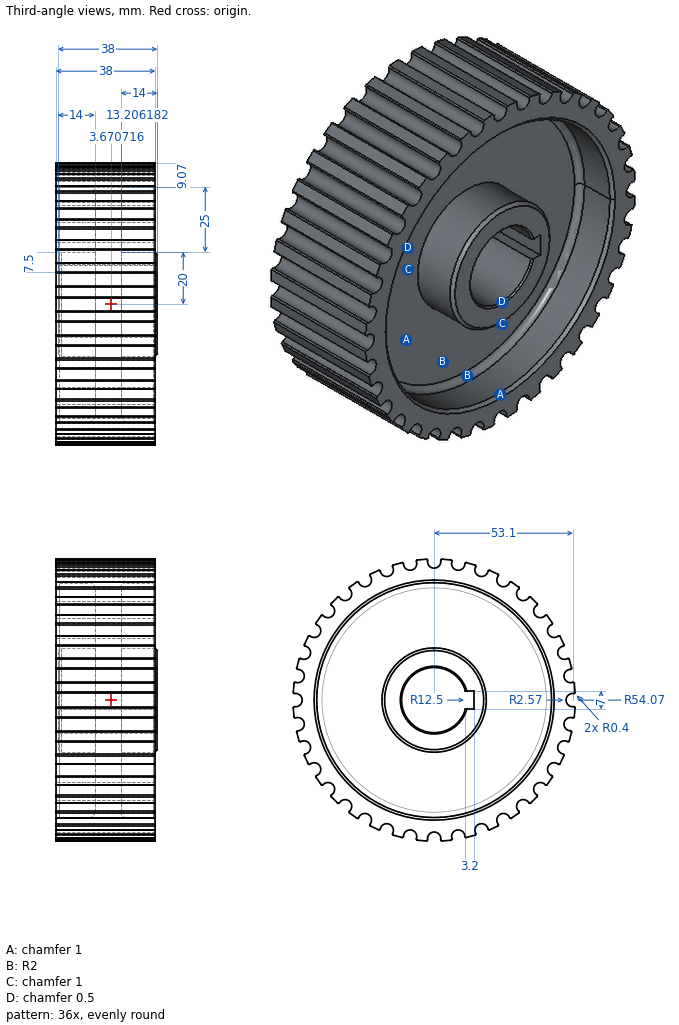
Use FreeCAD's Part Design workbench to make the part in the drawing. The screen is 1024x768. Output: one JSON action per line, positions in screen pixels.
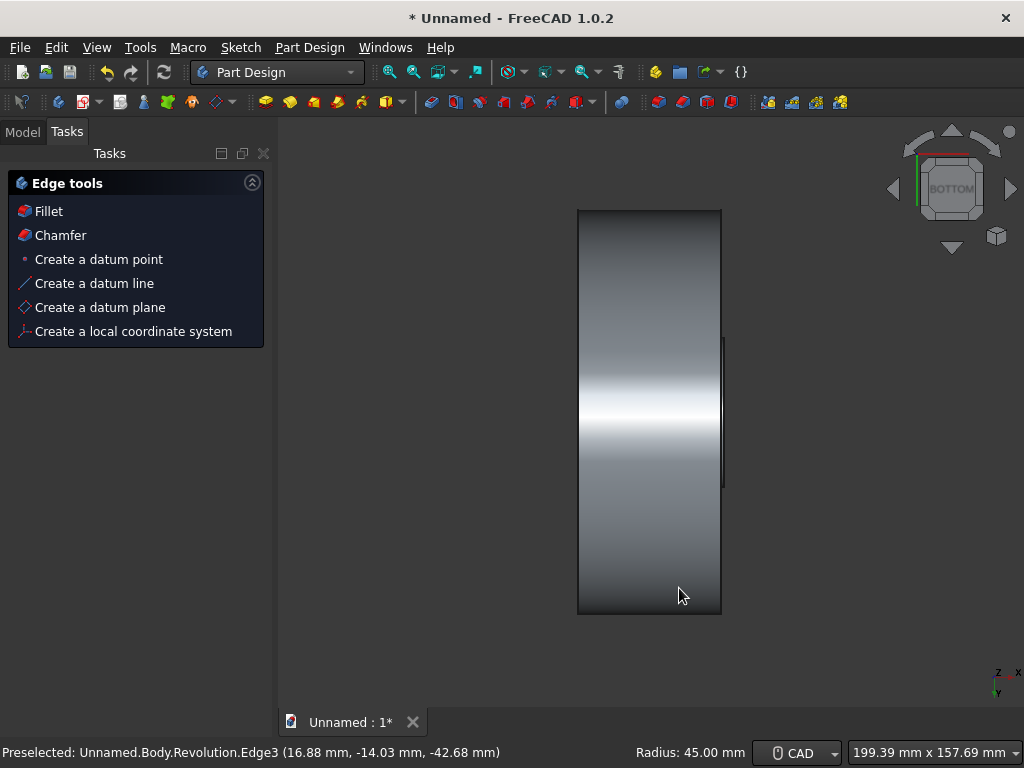
{"action": "key", "text": "4"}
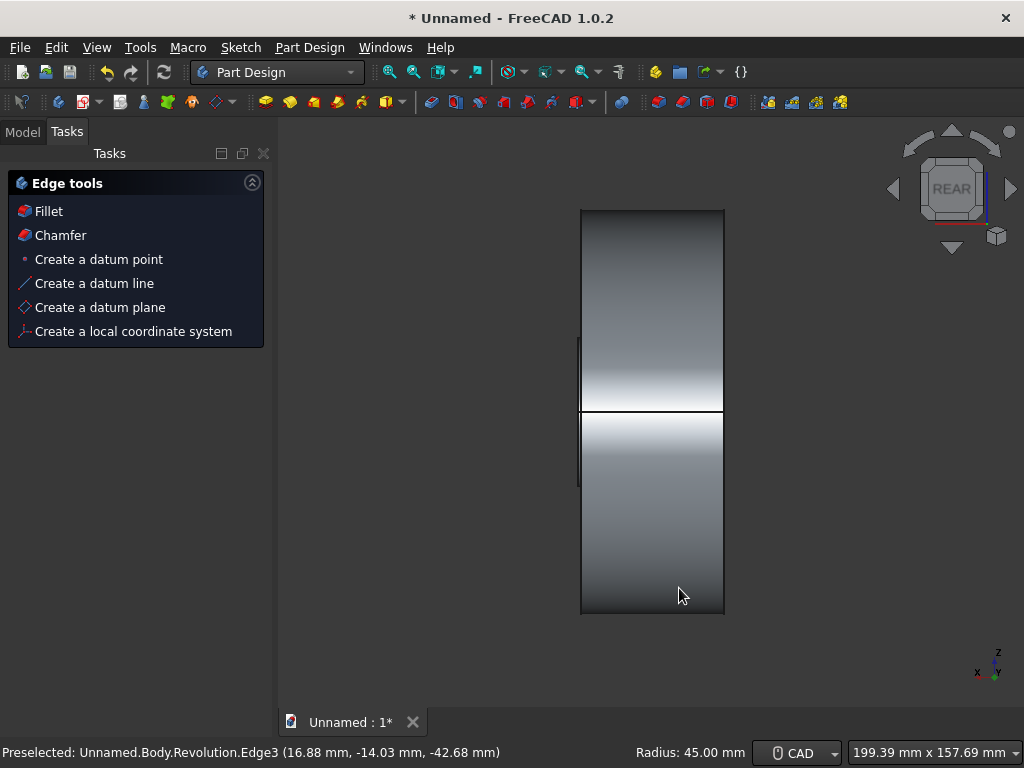
{"action": "key", "text": "6"}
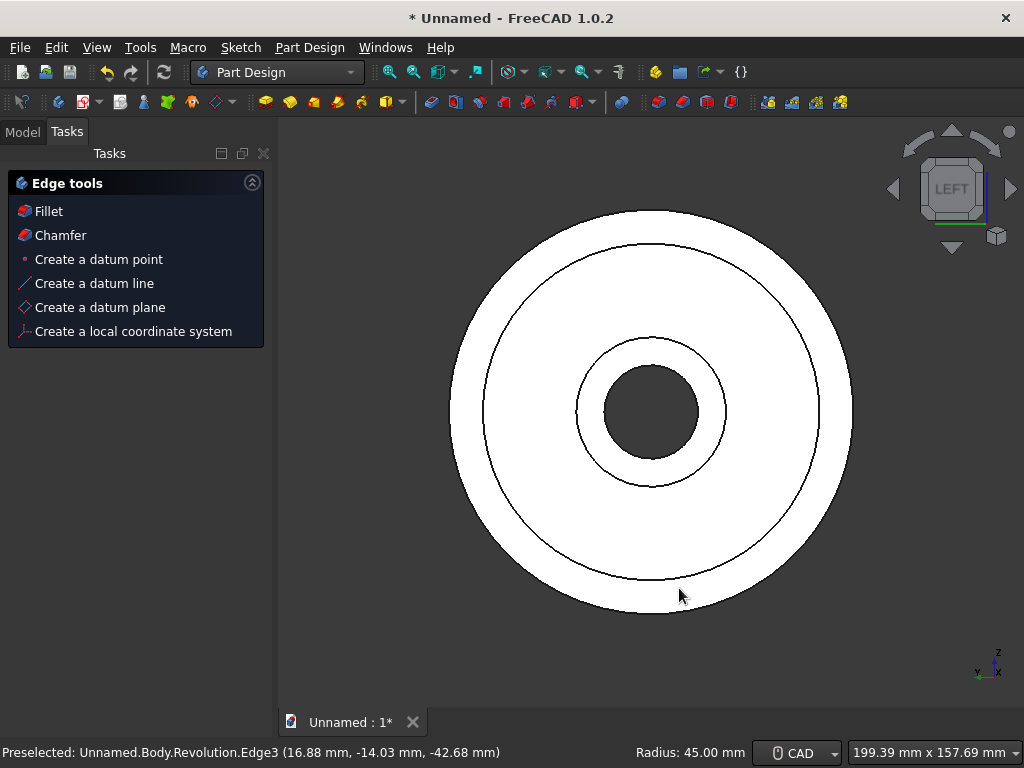
{"action": "left_click", "coordinate": [820, 411], "text": "ctrl"}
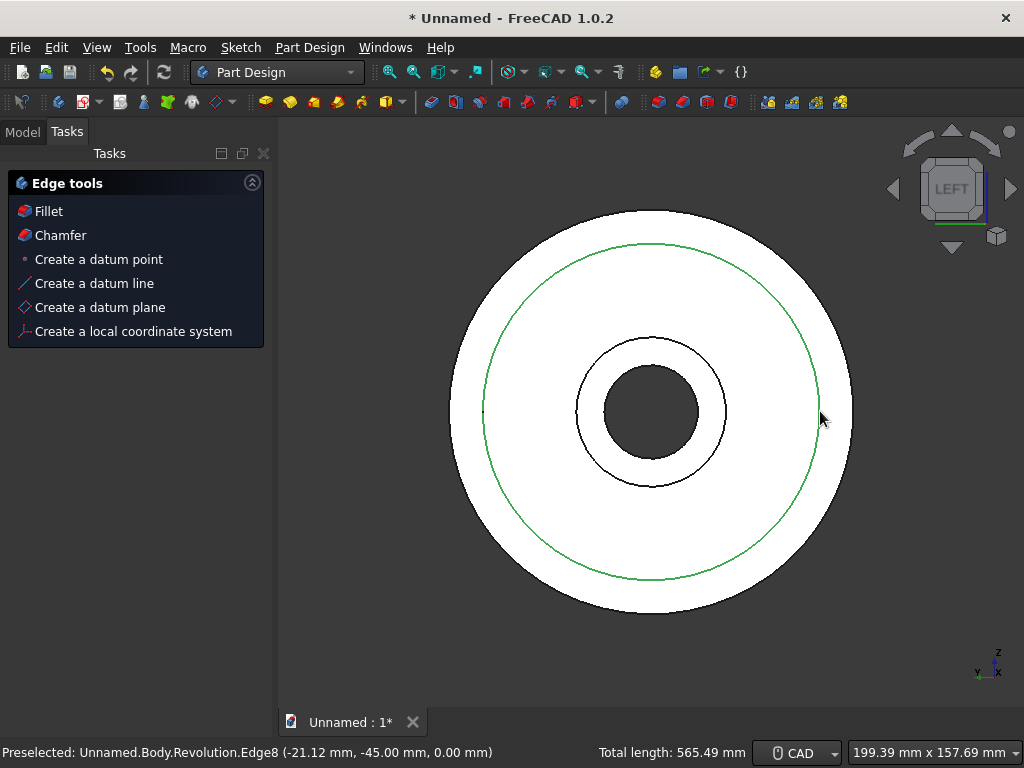
{"action": "left_click", "coordinate": [684, 102]}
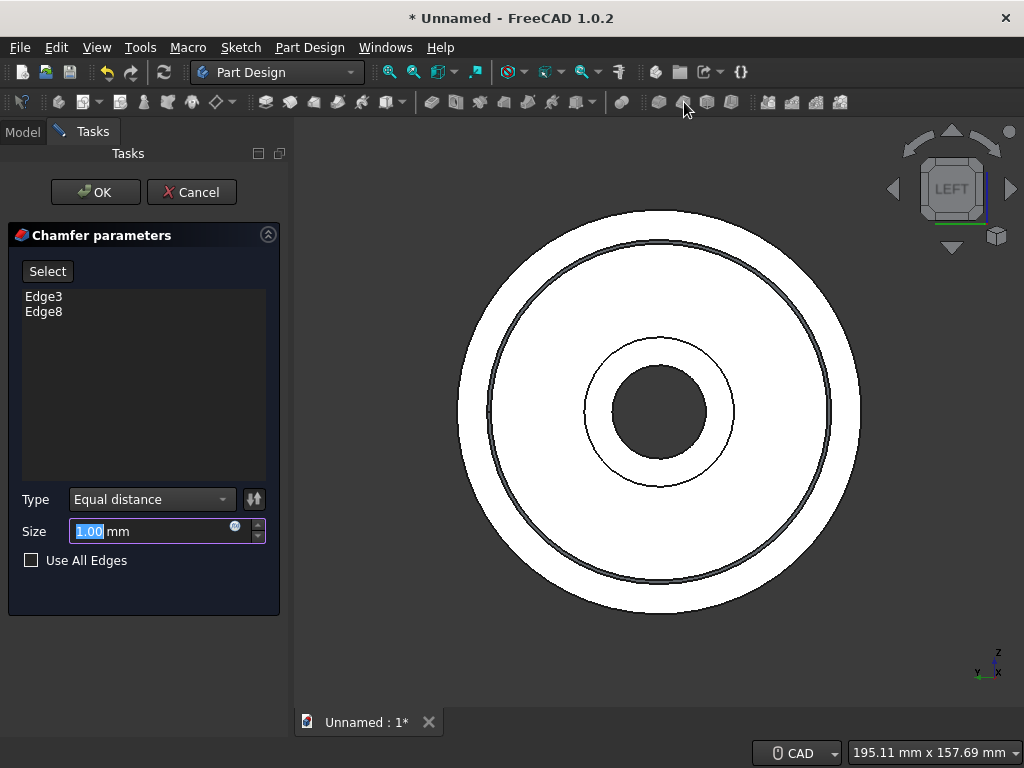
{"action": "type", "text": "1"}
{"action": "key", "text": "Tab"}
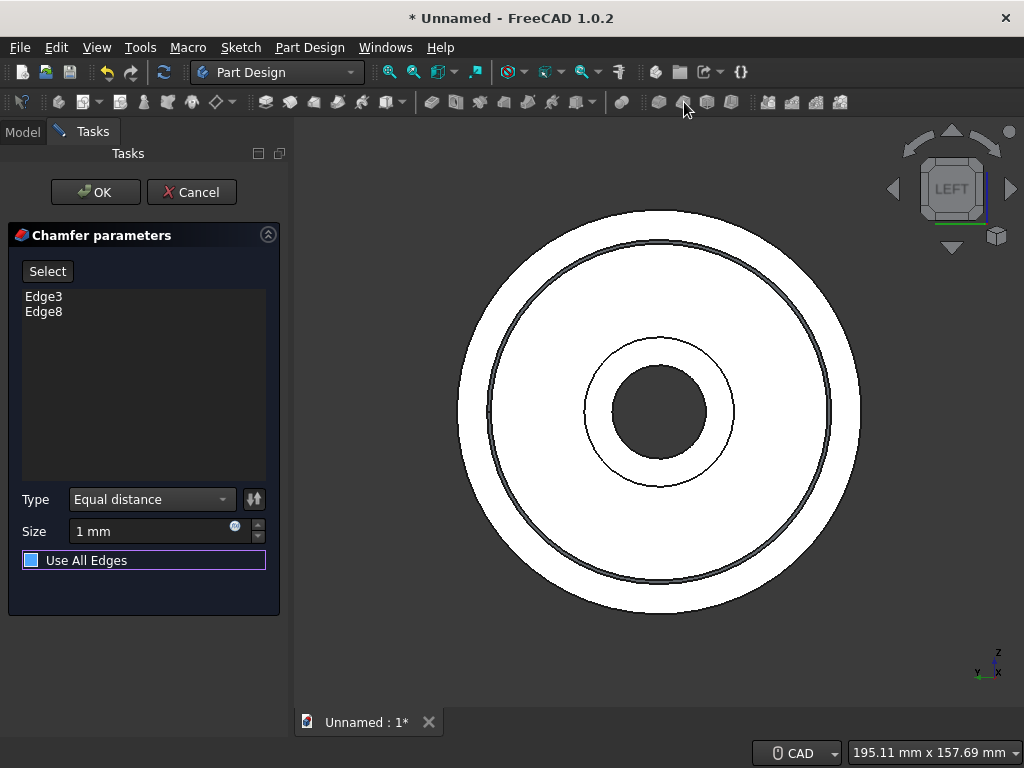
{"action": "left_click", "coordinate": [96, 192]}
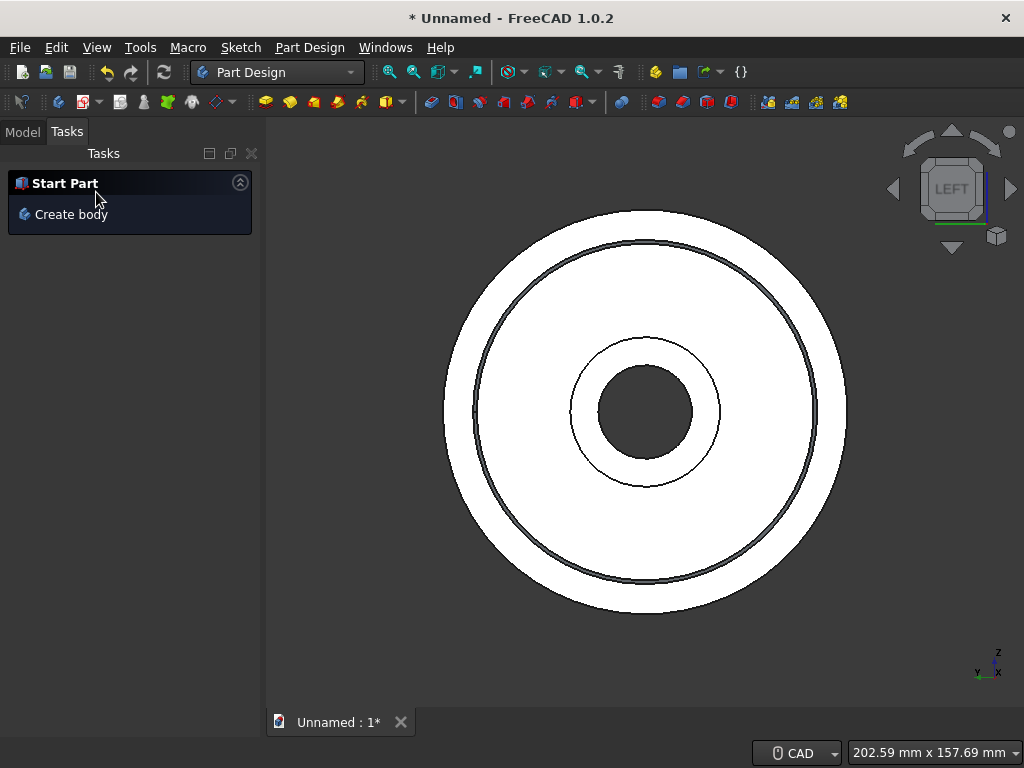
{"action": "key", "text": "0"}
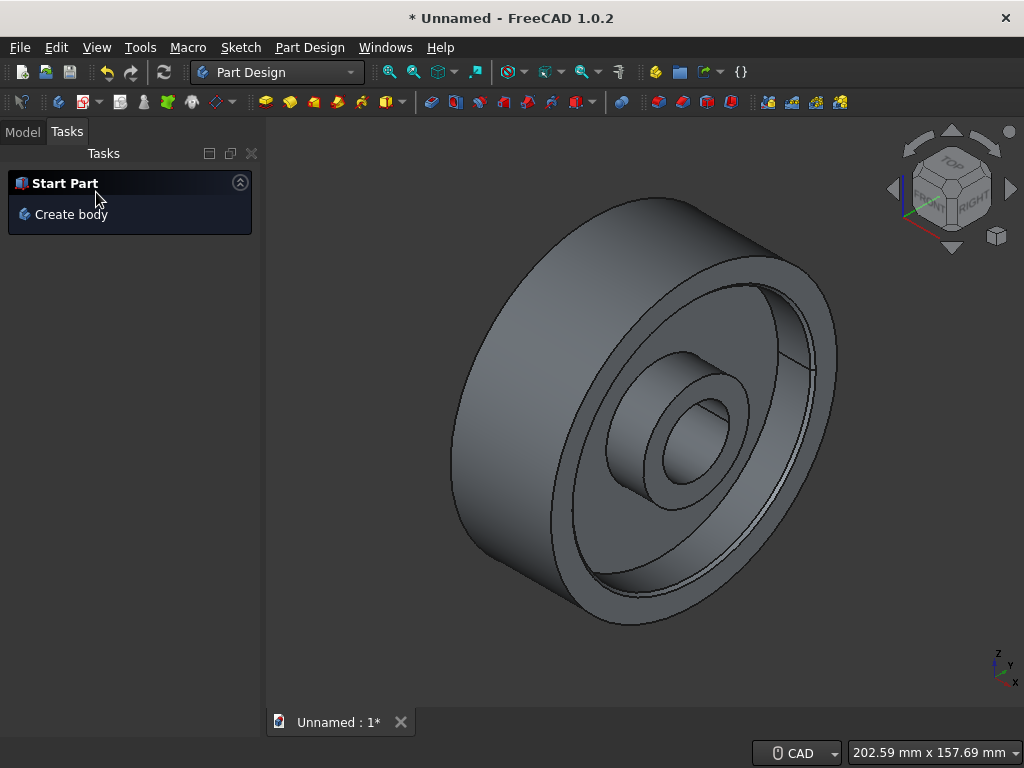
{"action": "key", "text": "2"}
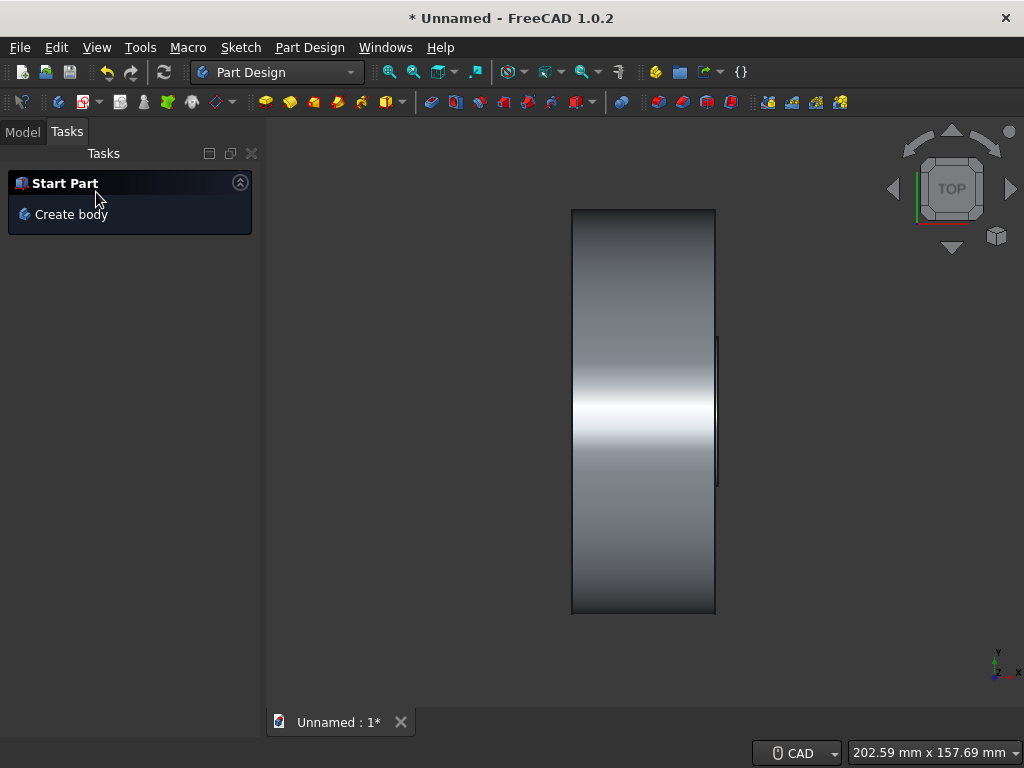
{"action": "key", "text": "1"}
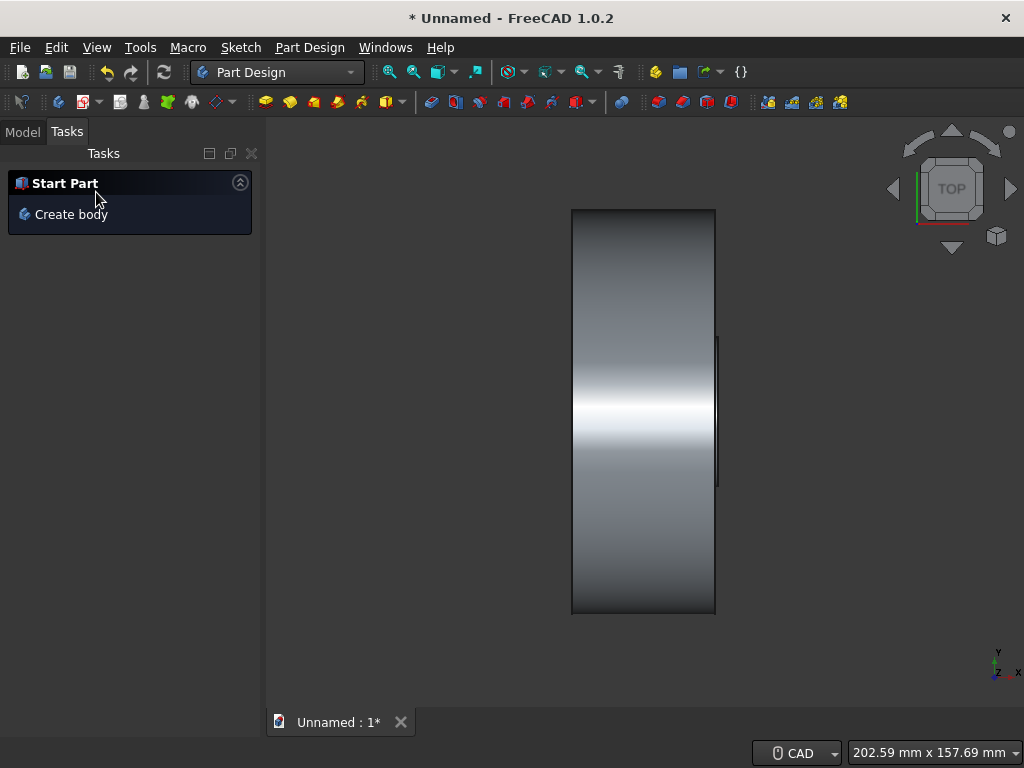
{"action": "key", "text": "3"}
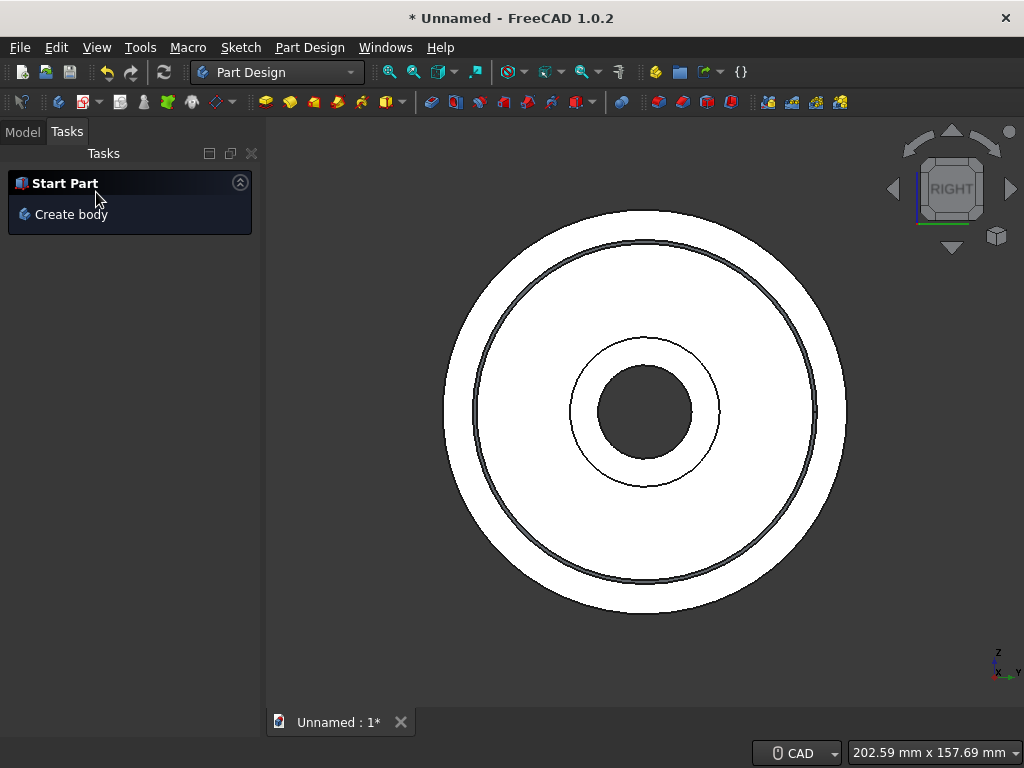
{"action": "key", "text": "5"}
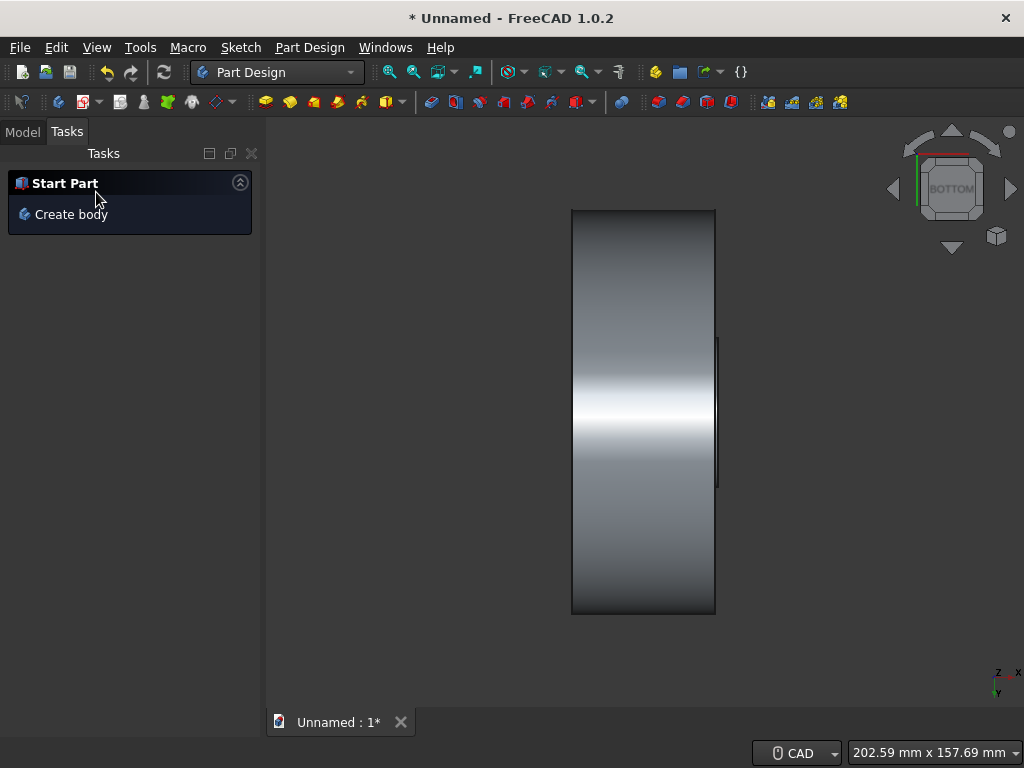
{"action": "key", "text": "4"}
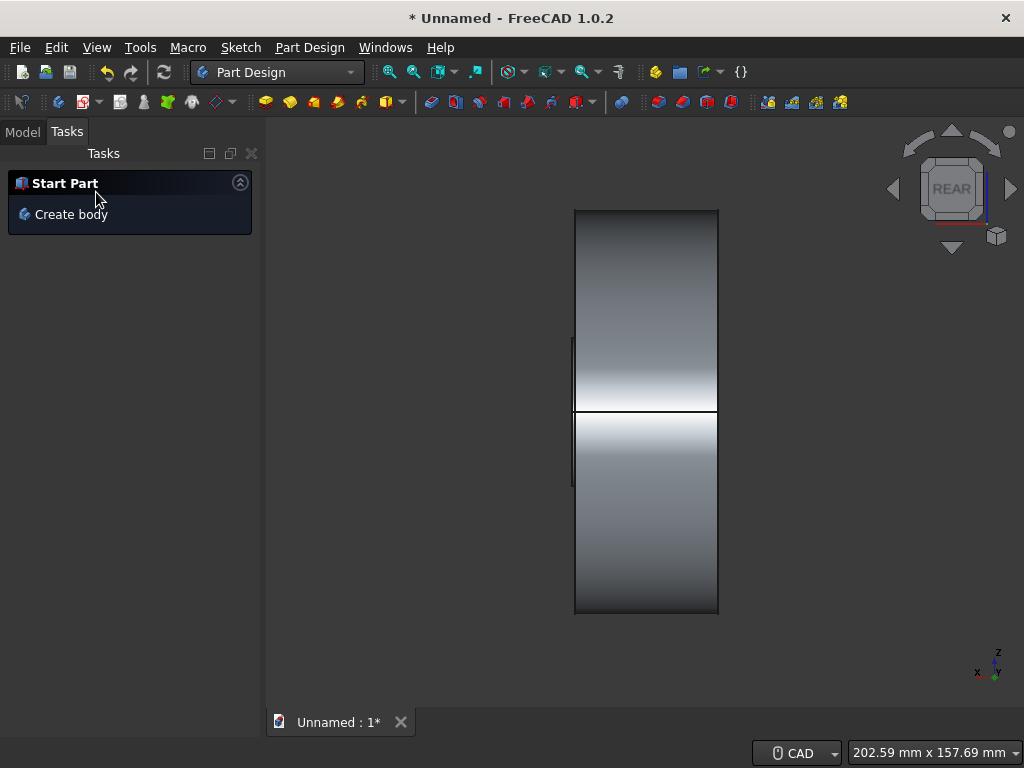
{"action": "key", "text": "6"}